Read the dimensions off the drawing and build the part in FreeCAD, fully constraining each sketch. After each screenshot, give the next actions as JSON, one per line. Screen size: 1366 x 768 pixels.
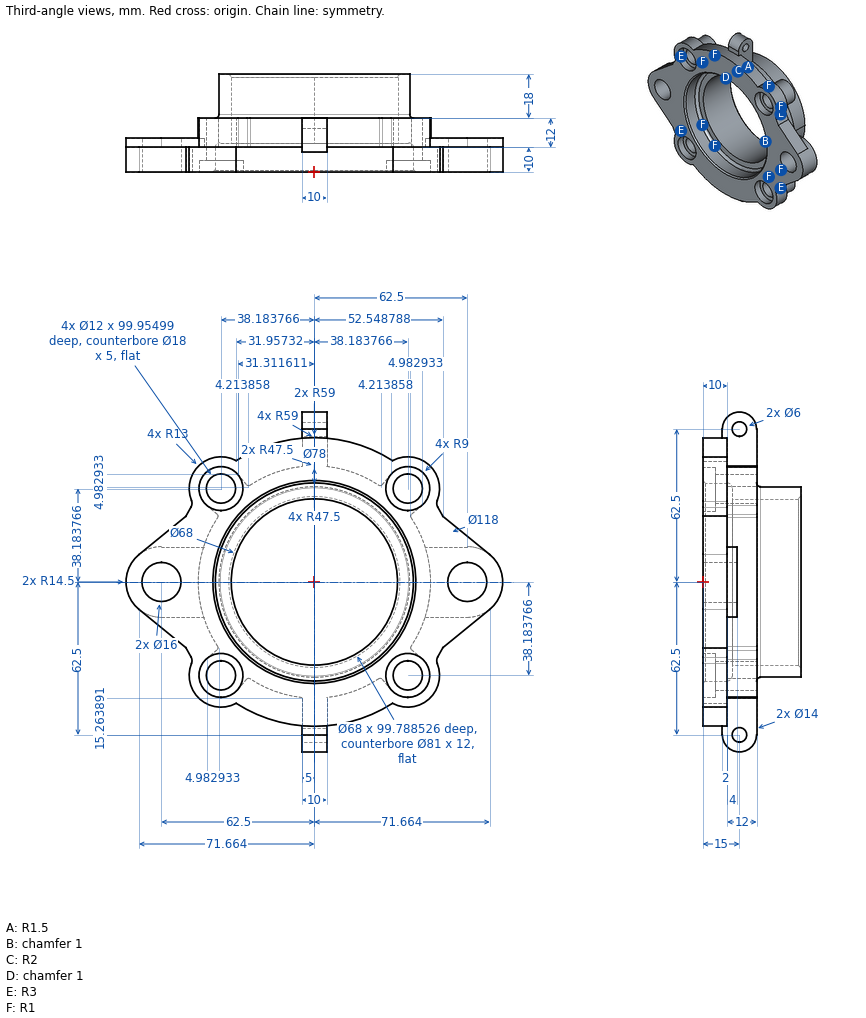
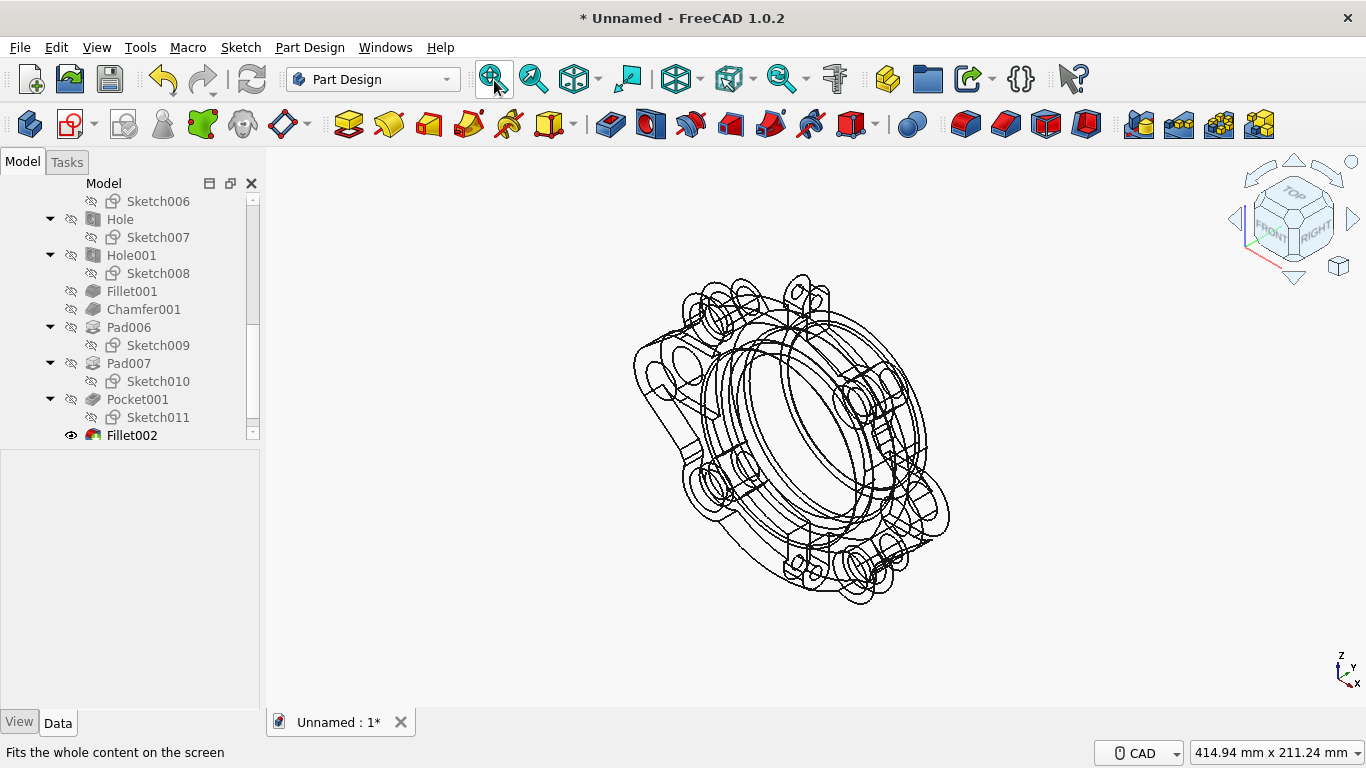
{"action": "left_click", "coordinate": [864, 542]}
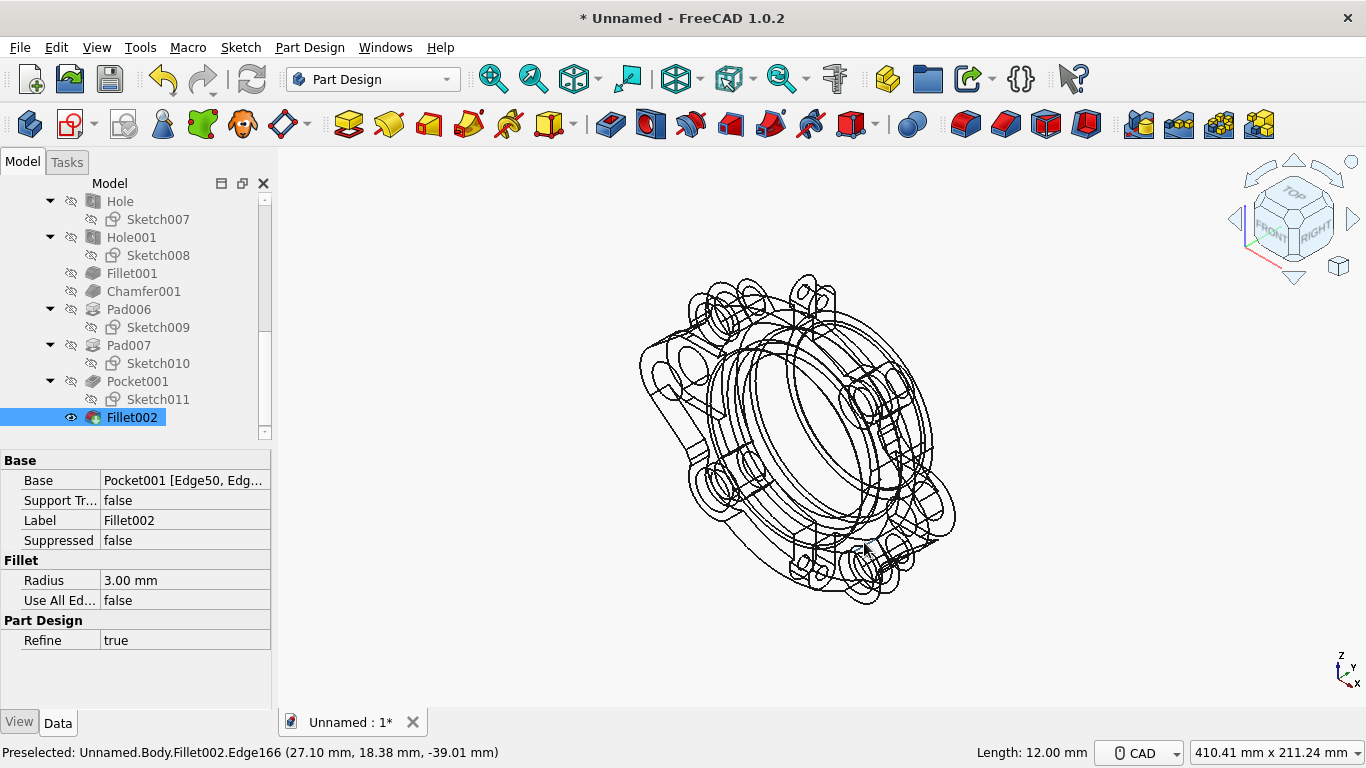
{"action": "left_click", "coordinate": [746, 327], "text": "ctrl"}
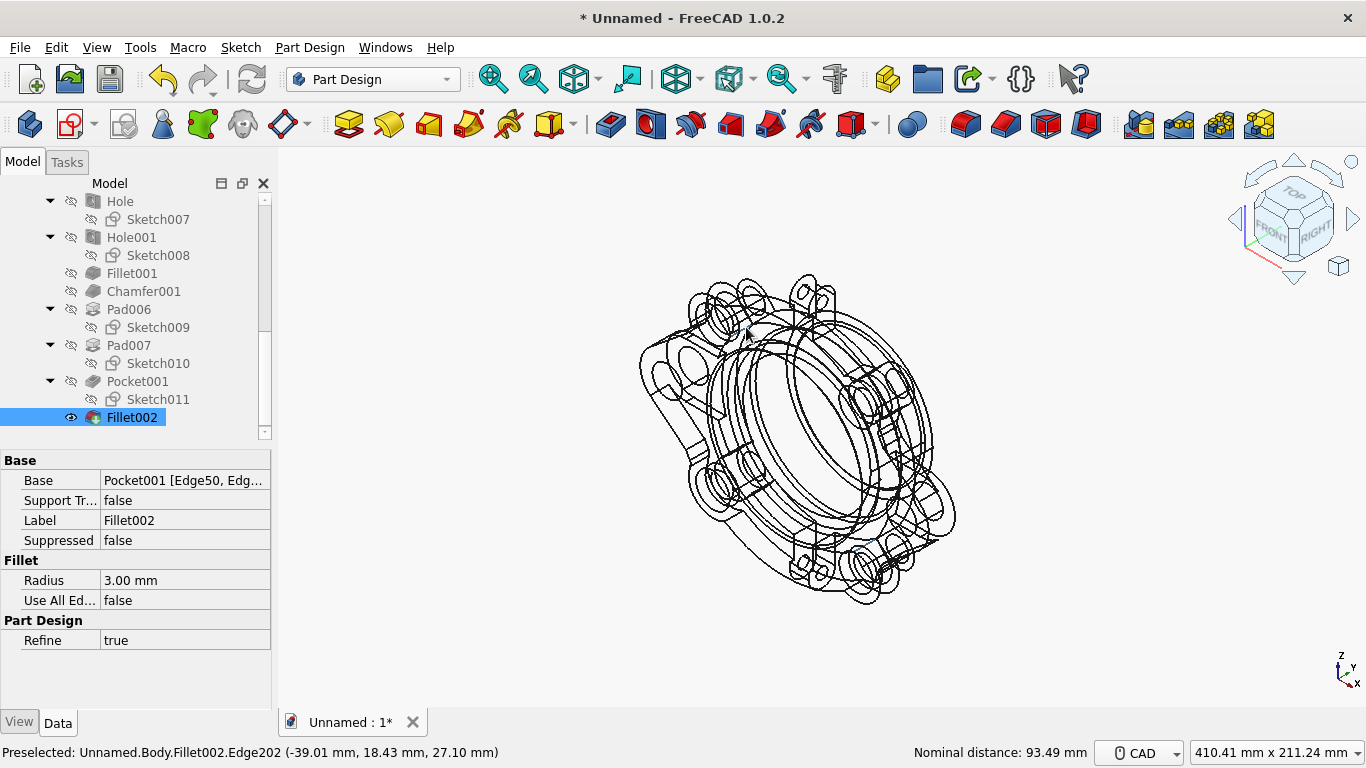
{"action": "key", "text": "2"}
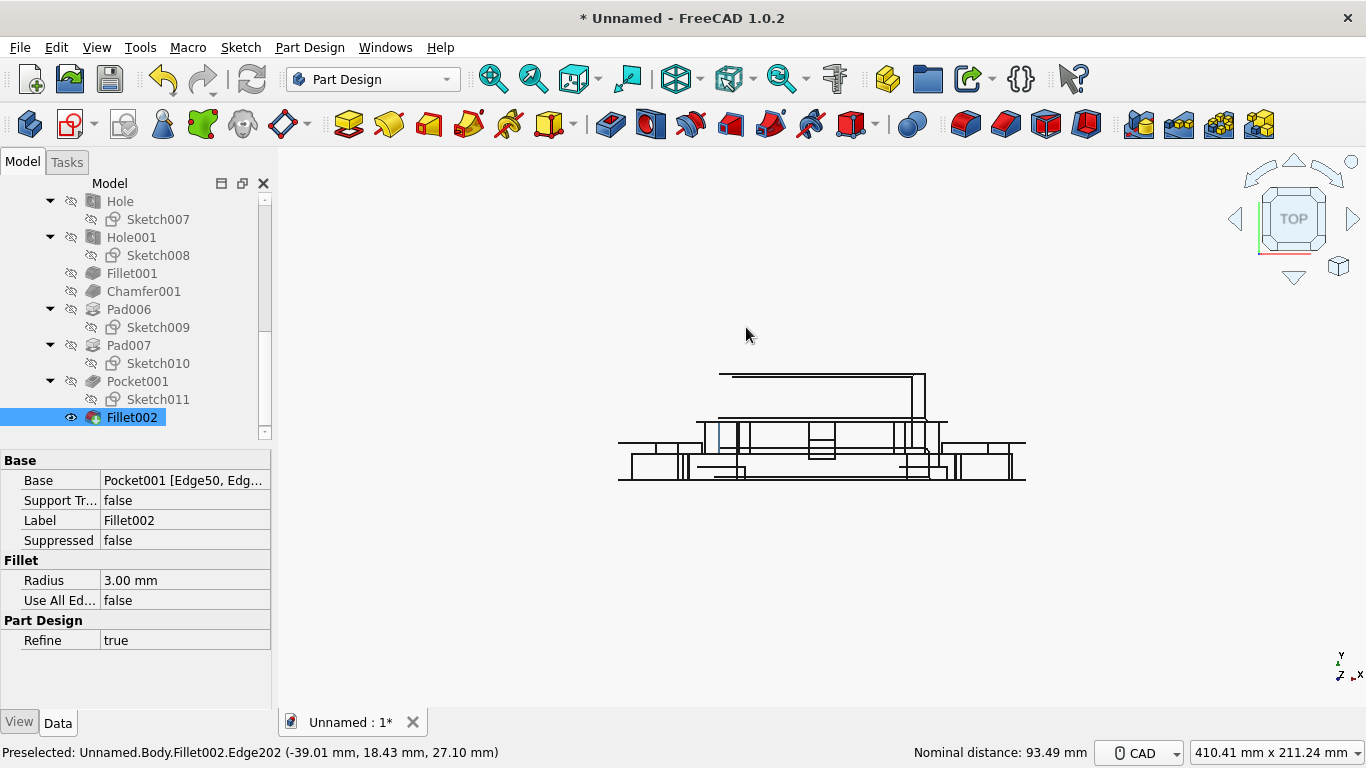
{"action": "left_click", "coordinate": [494, 80]}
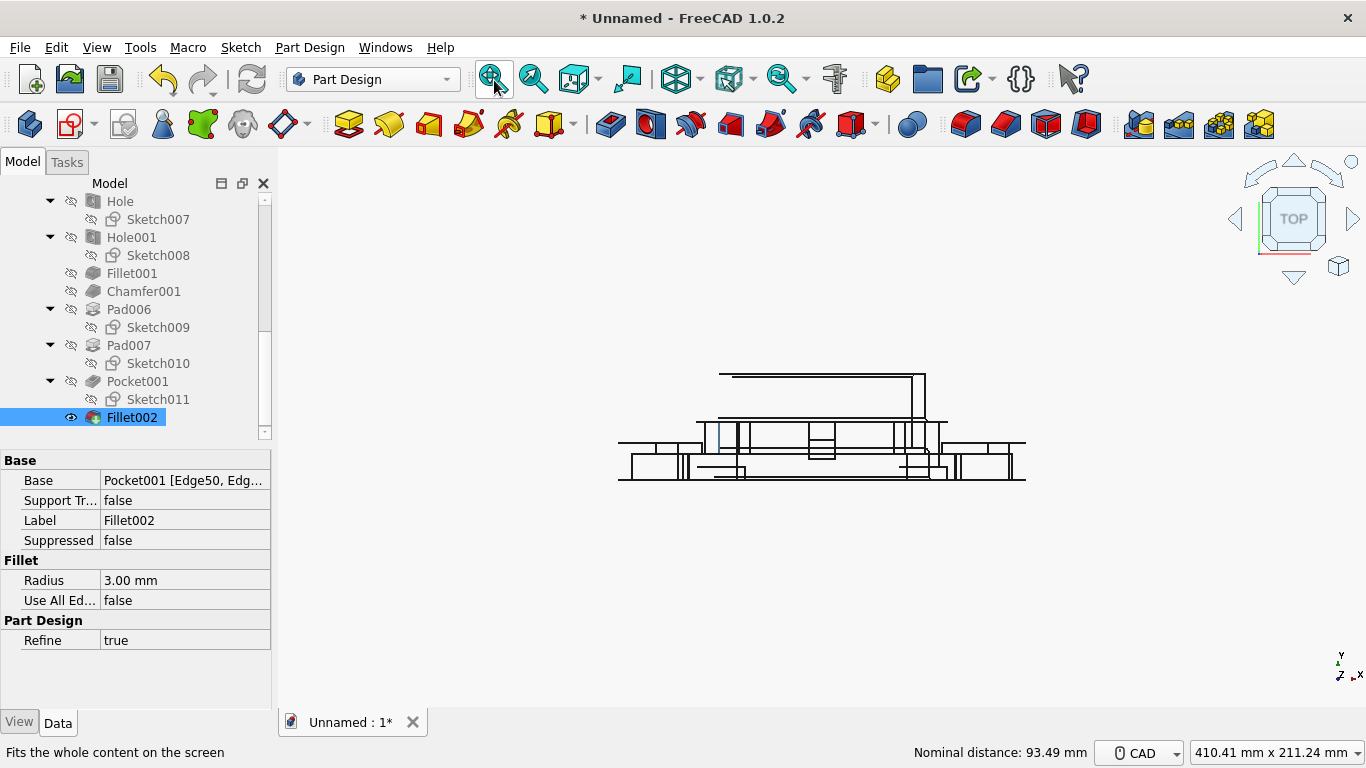
{"action": "left_click", "coordinate": [750, 437], "text": "ctrl"}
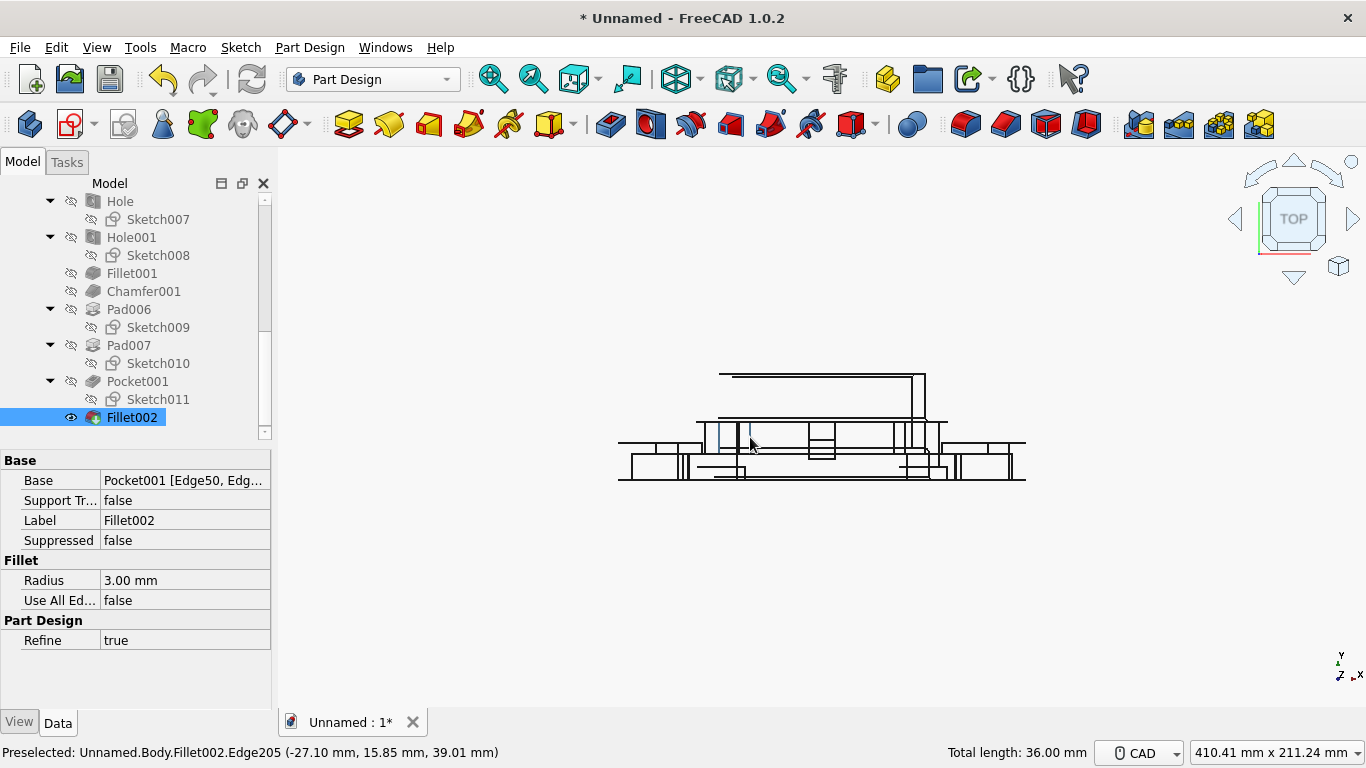
{"action": "left_click", "coordinate": [894, 437], "text": "ctrl"}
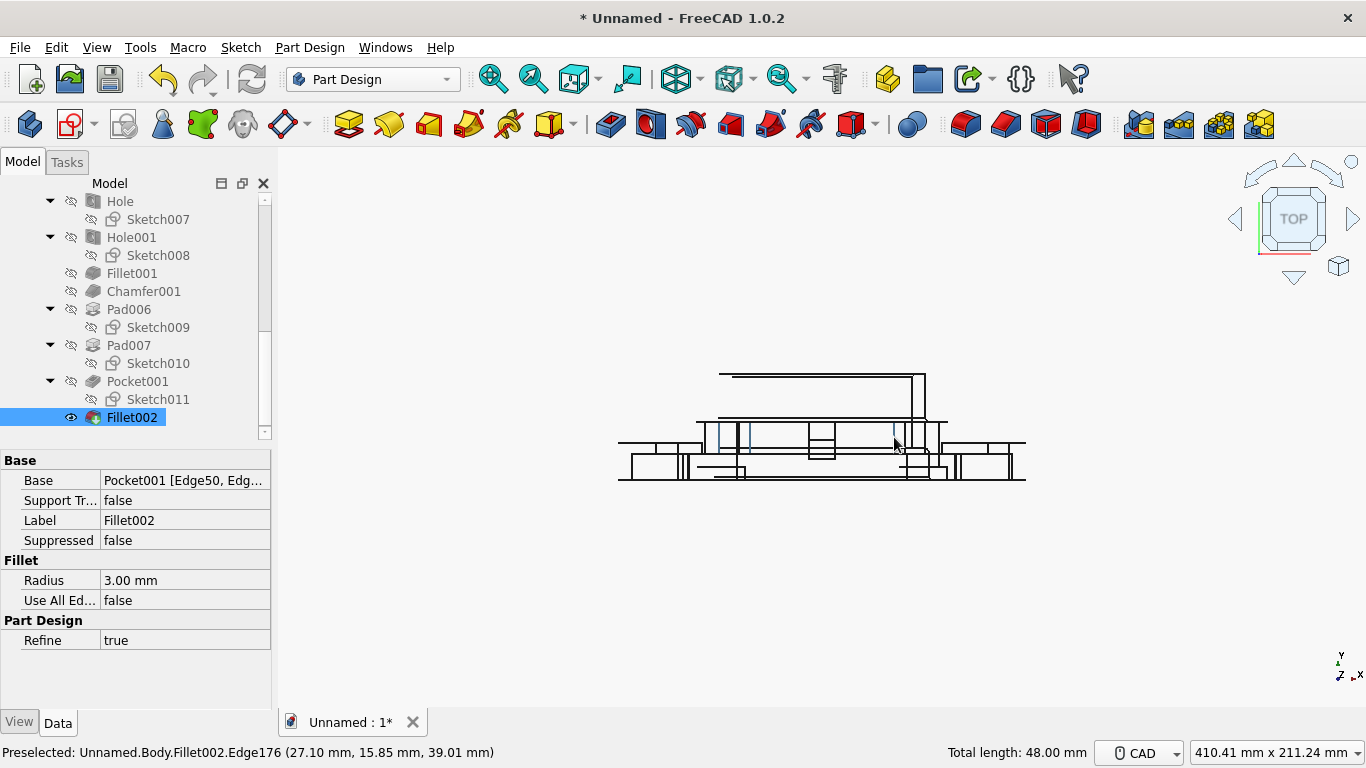
{"action": "left_click", "coordinate": [925, 437], "text": "ctrl"}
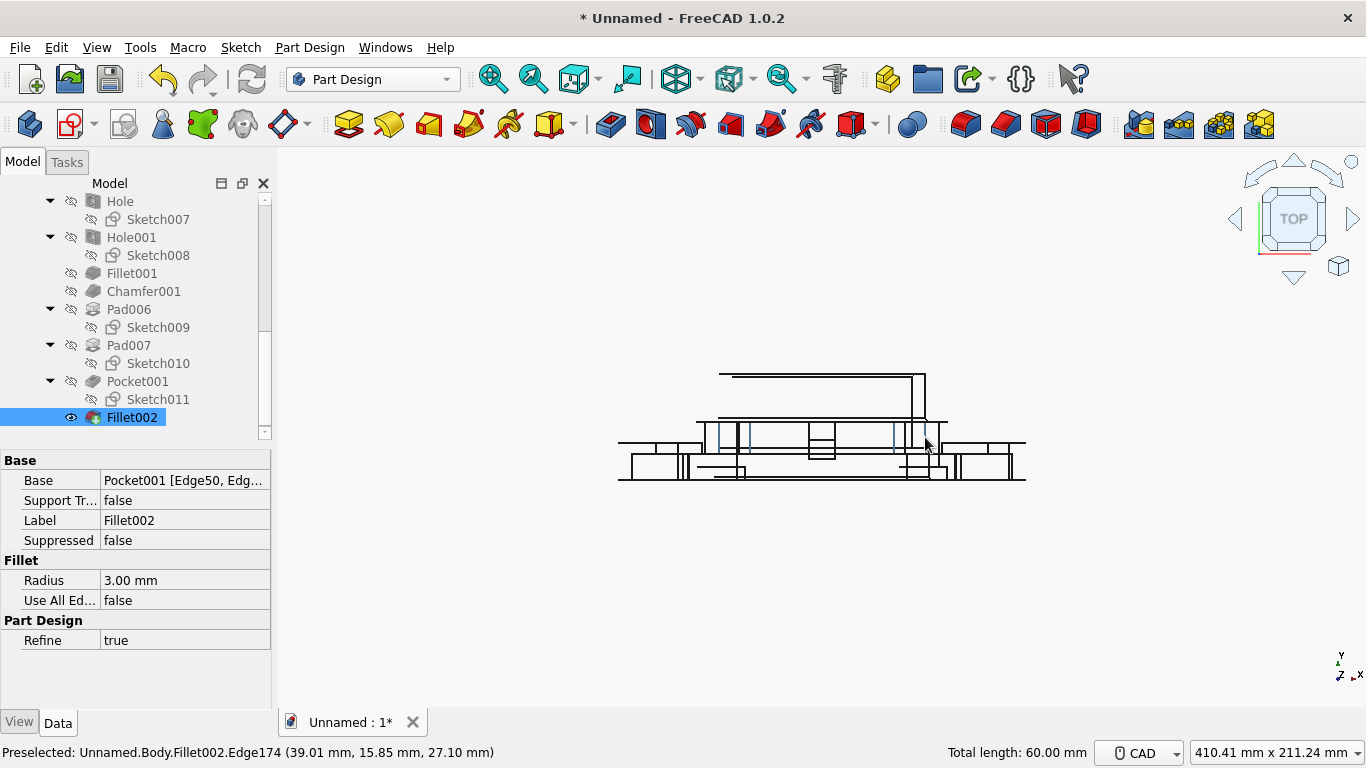
{"action": "key", "text": "1"}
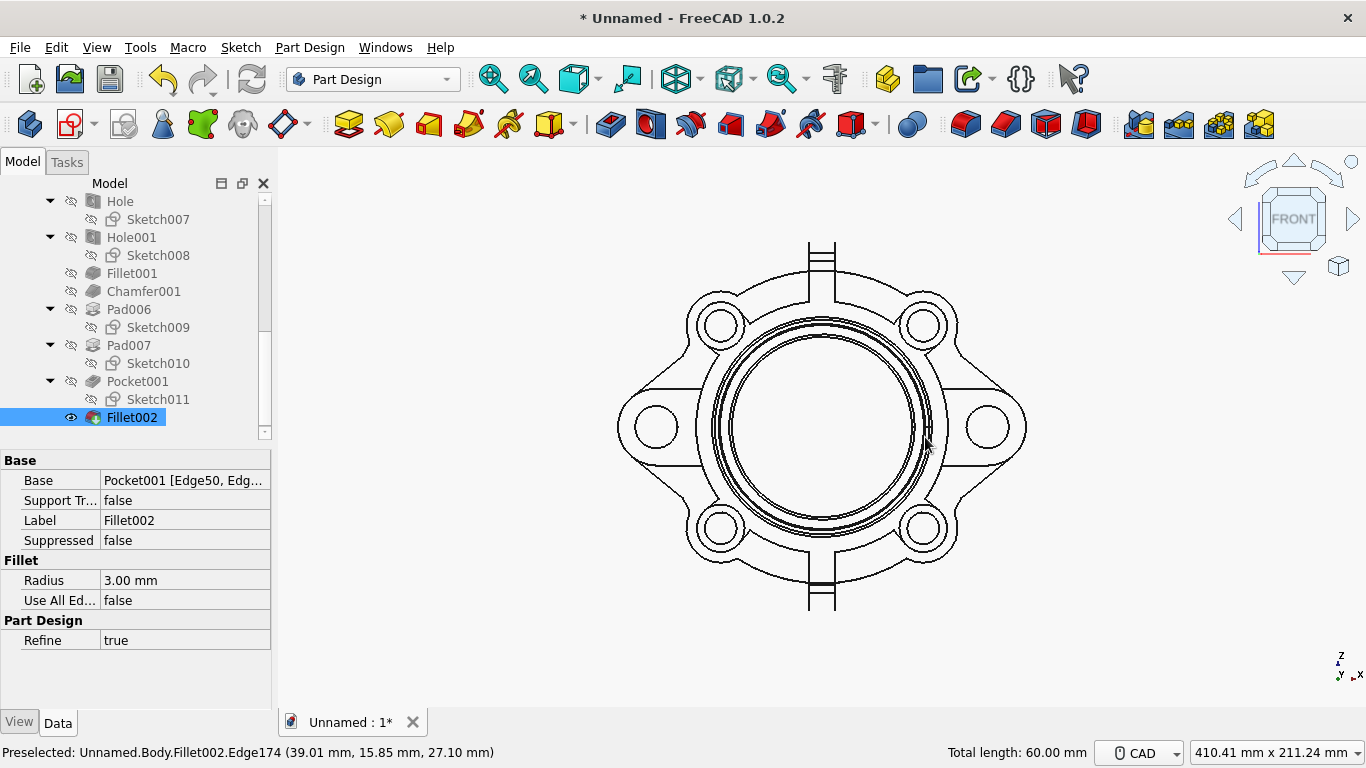
{"action": "key", "text": "3"}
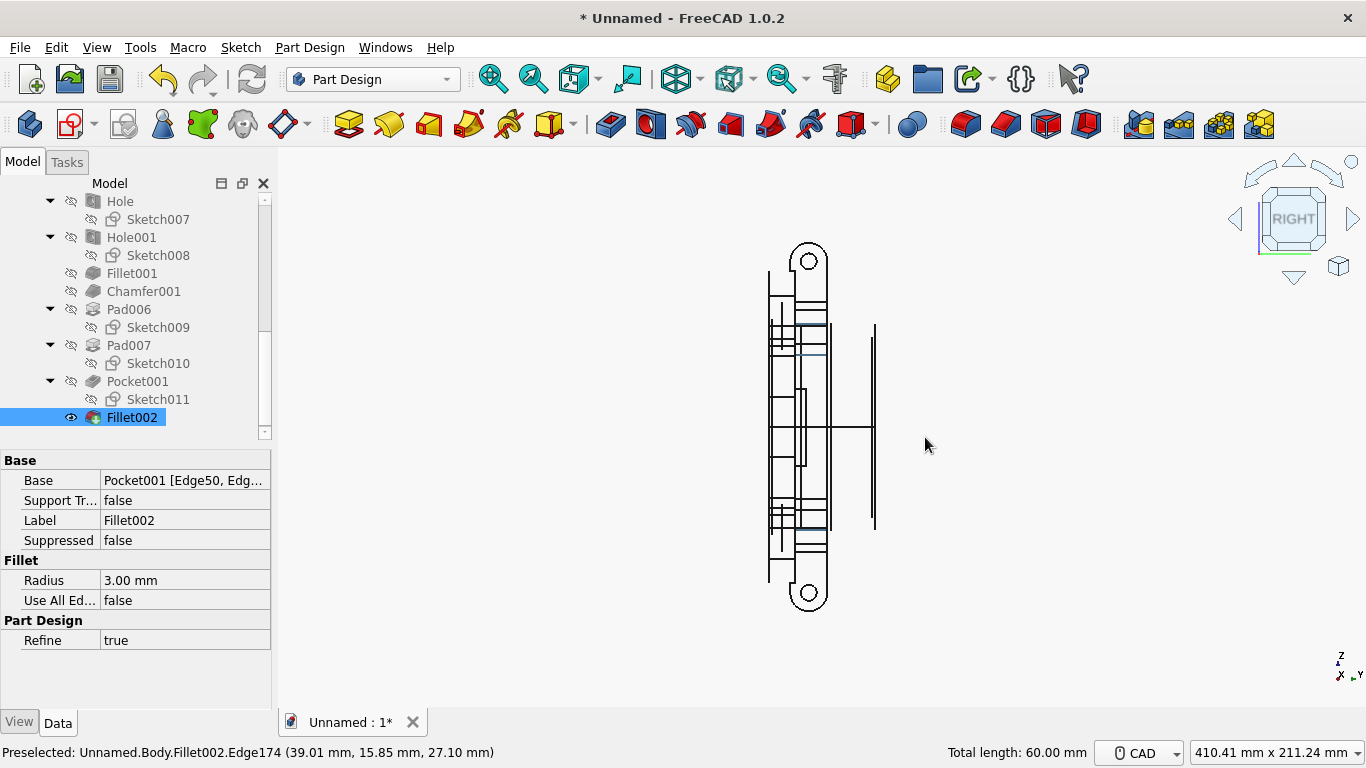
{"action": "left_click", "coordinate": [811, 498], "text": "ctrl"}